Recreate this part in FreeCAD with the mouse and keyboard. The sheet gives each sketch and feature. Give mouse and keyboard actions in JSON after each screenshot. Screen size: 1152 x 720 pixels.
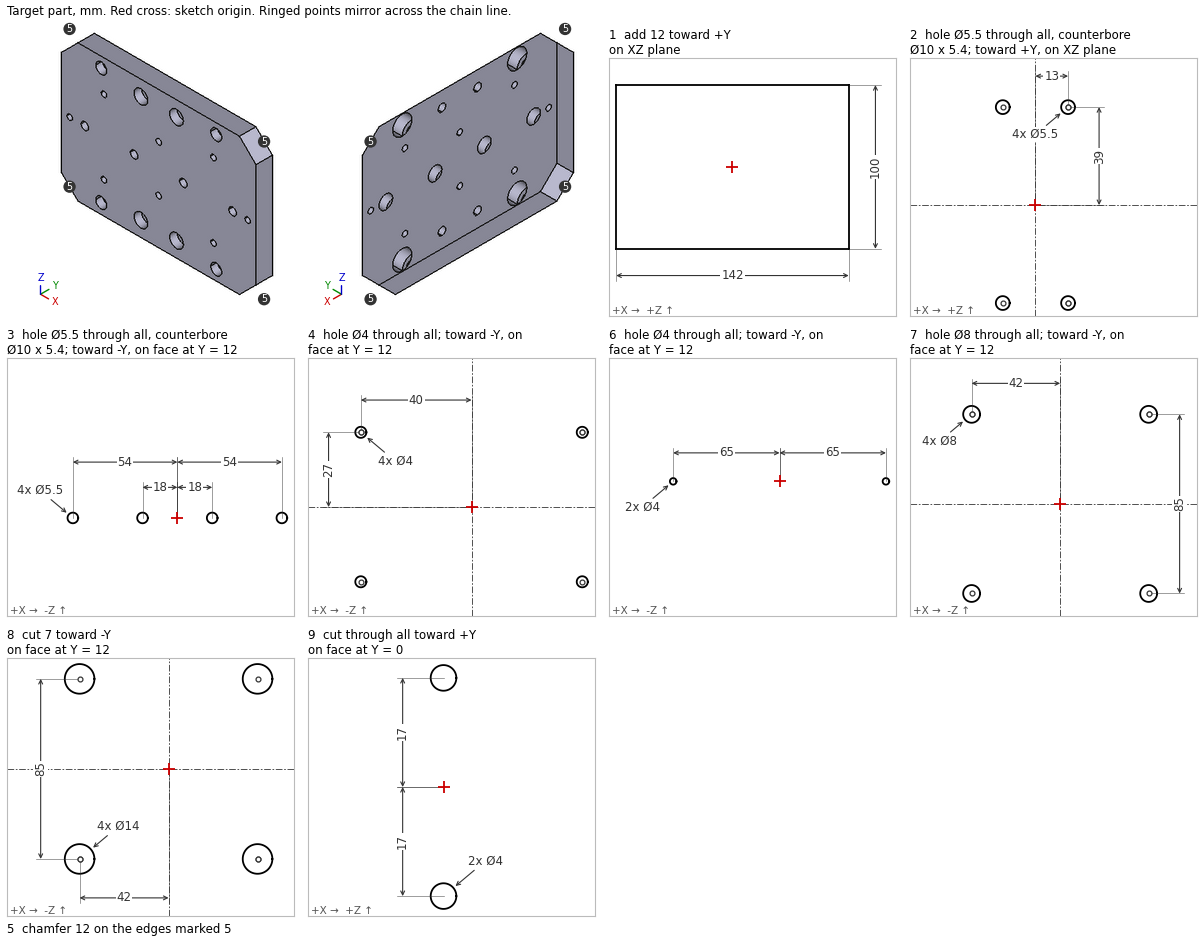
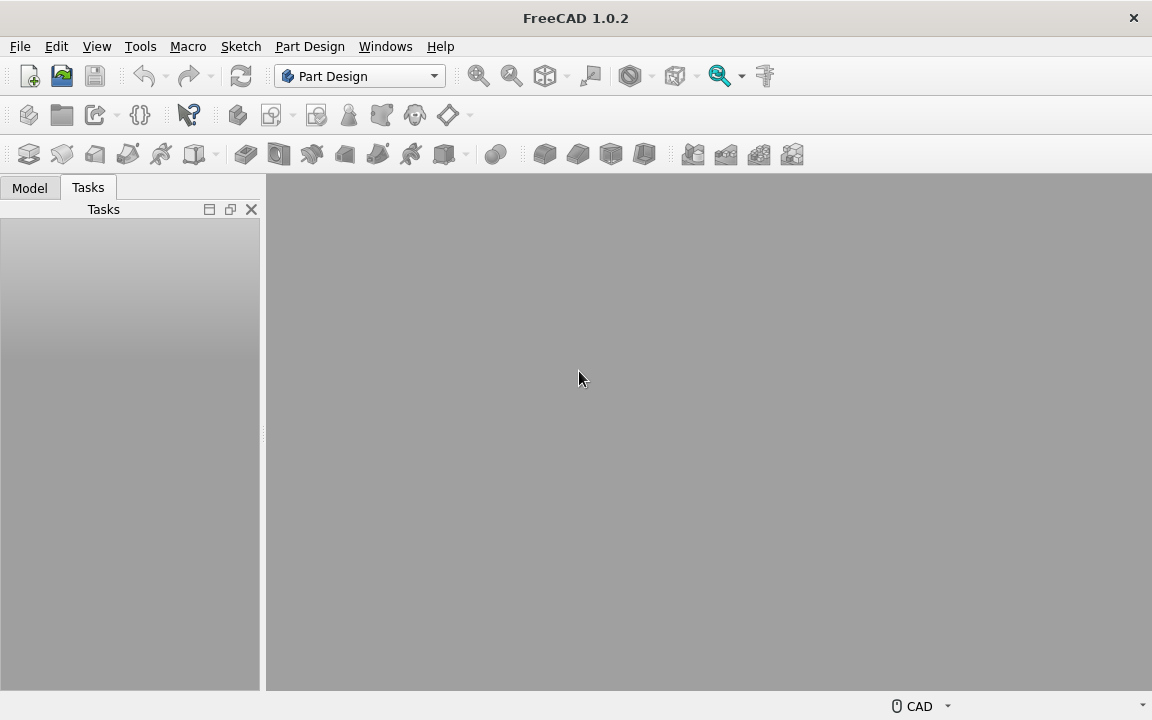
{"action": "left_click", "coordinate": [29, 76]}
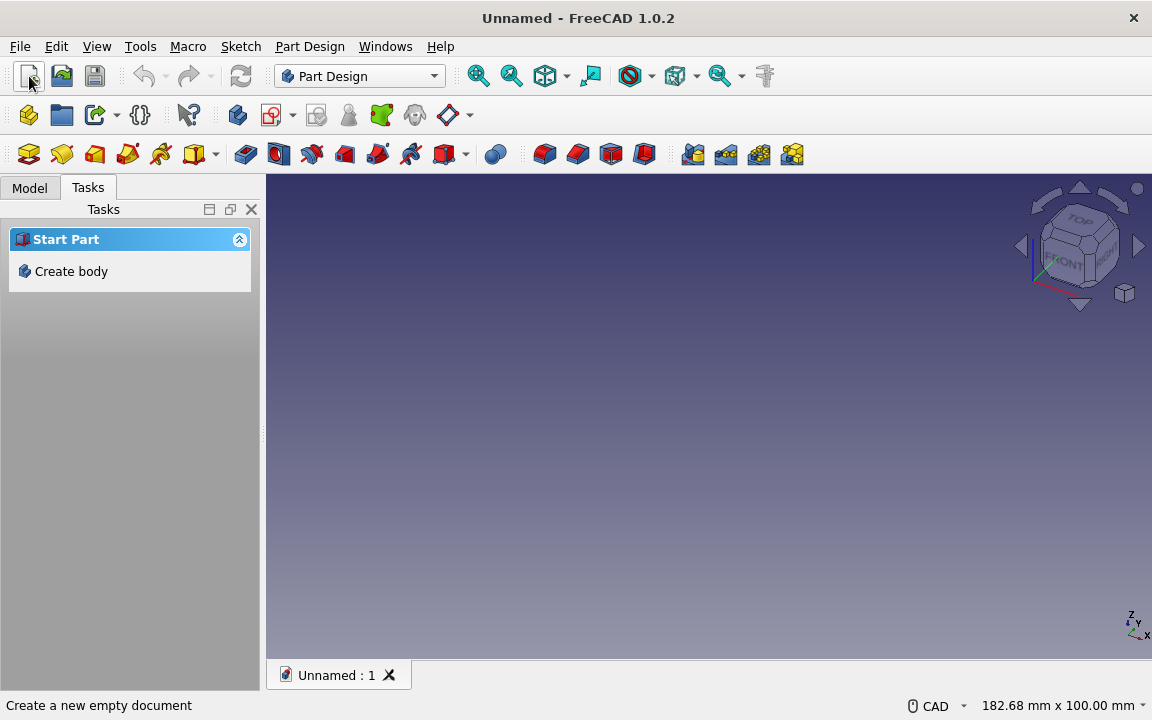
{"action": "left_click", "coordinate": [270, 116]}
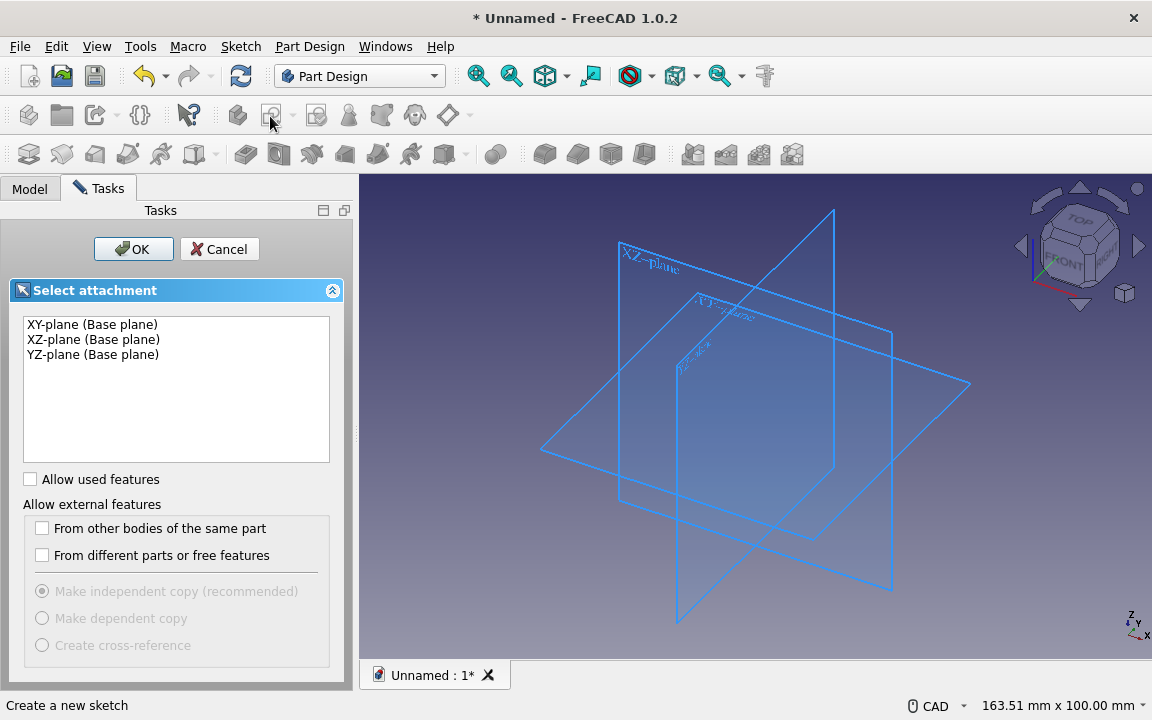
{"action": "left_click", "coordinate": [84, 340]}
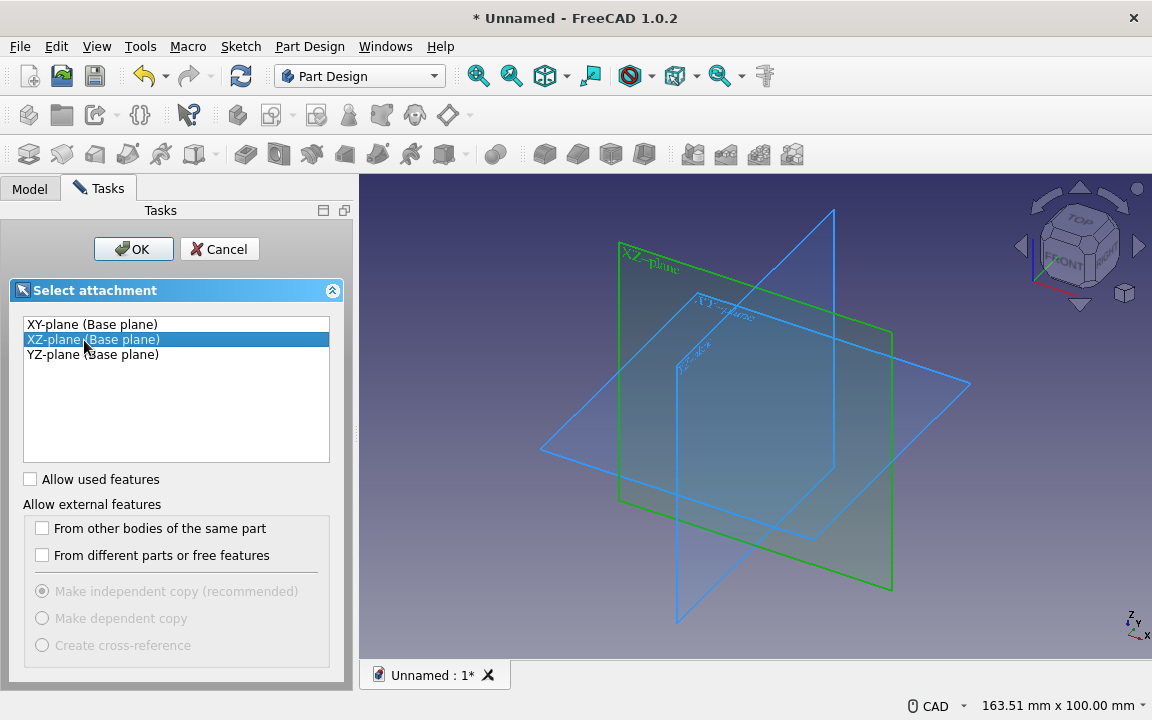
{"action": "left_click", "coordinate": [134, 249]}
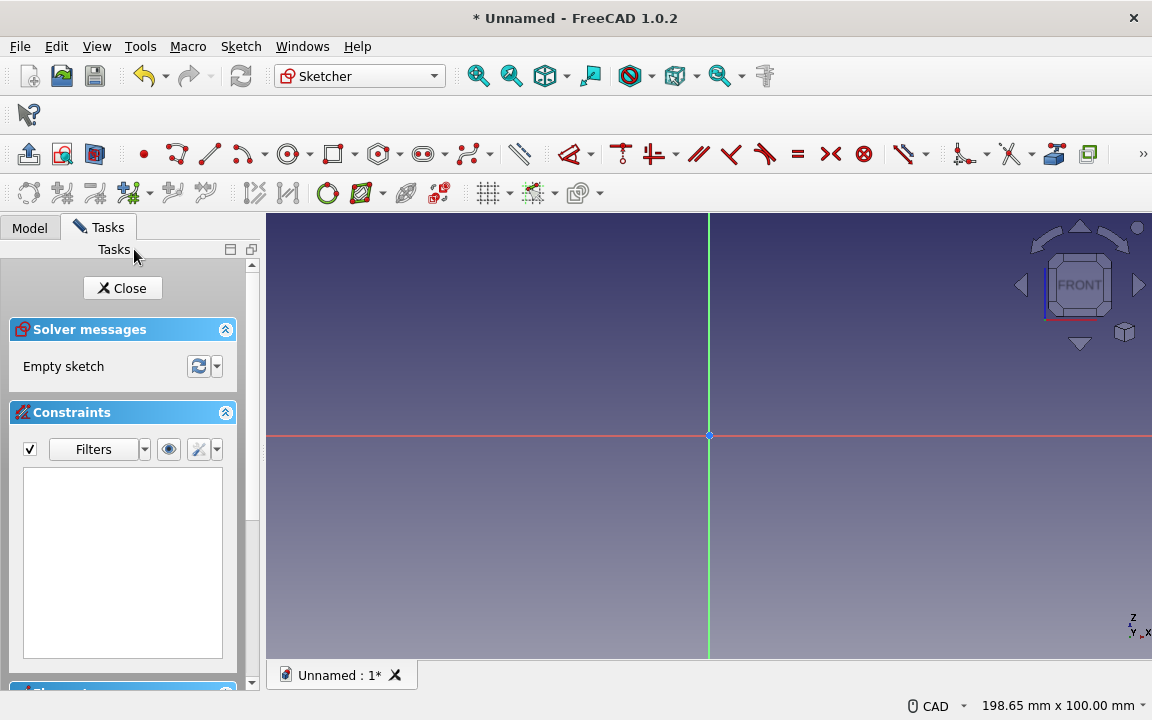
{"action": "scroll", "coordinate": [501, 436], "scroll_direction": "down", "scroll_amount": 2}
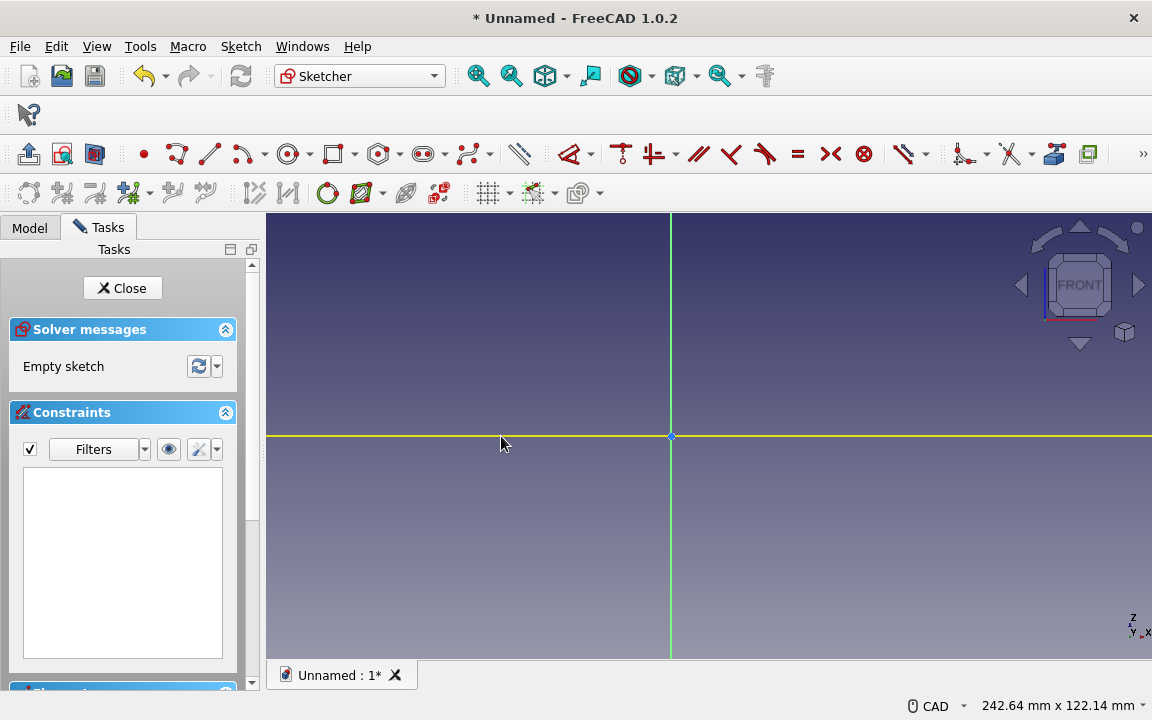
{"action": "left_click", "coordinate": [354, 154]}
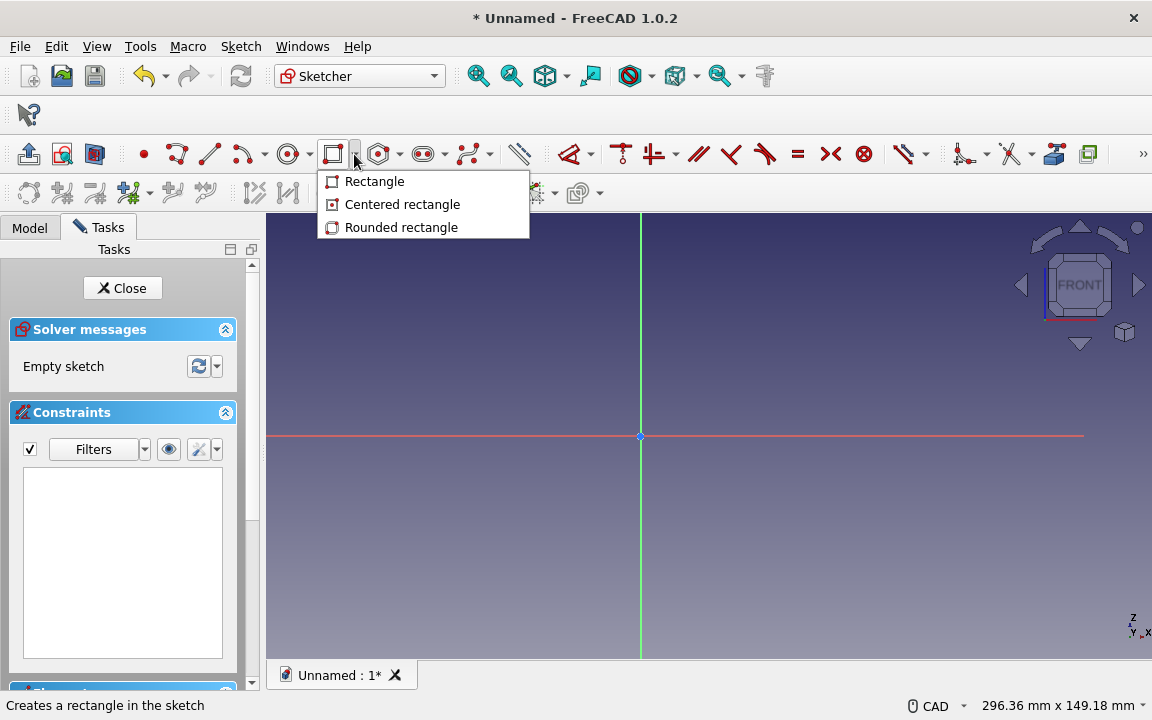
{"action": "left_click", "coordinate": [424, 204]}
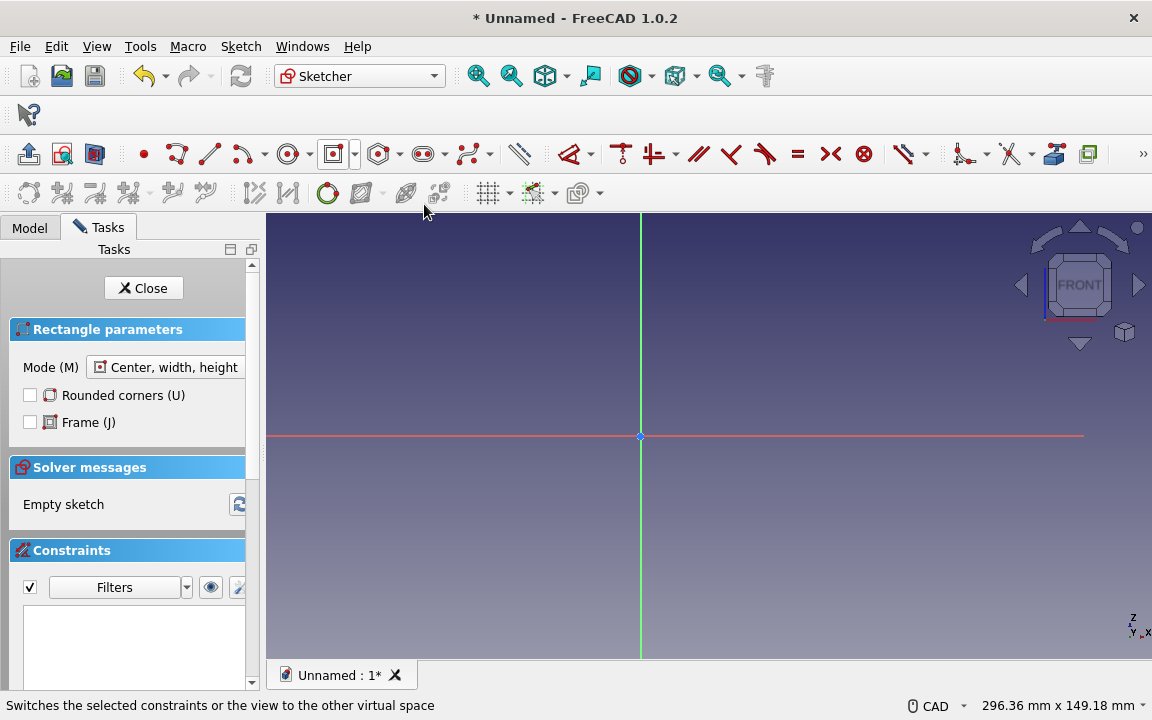
{"action": "left_click", "coordinate": [641, 436]}
{"action": "left_click", "coordinate": [853, 287]}
{"action": "key", "text": "Escape"}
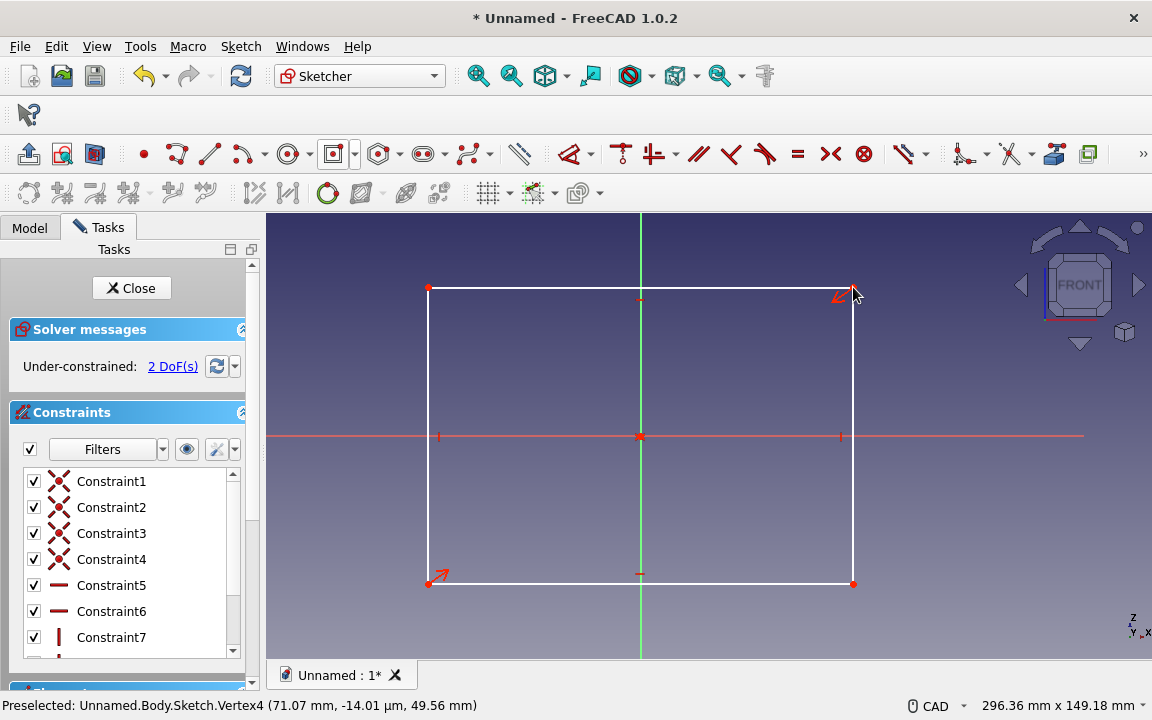
{"action": "left_click", "coordinate": [568, 154]}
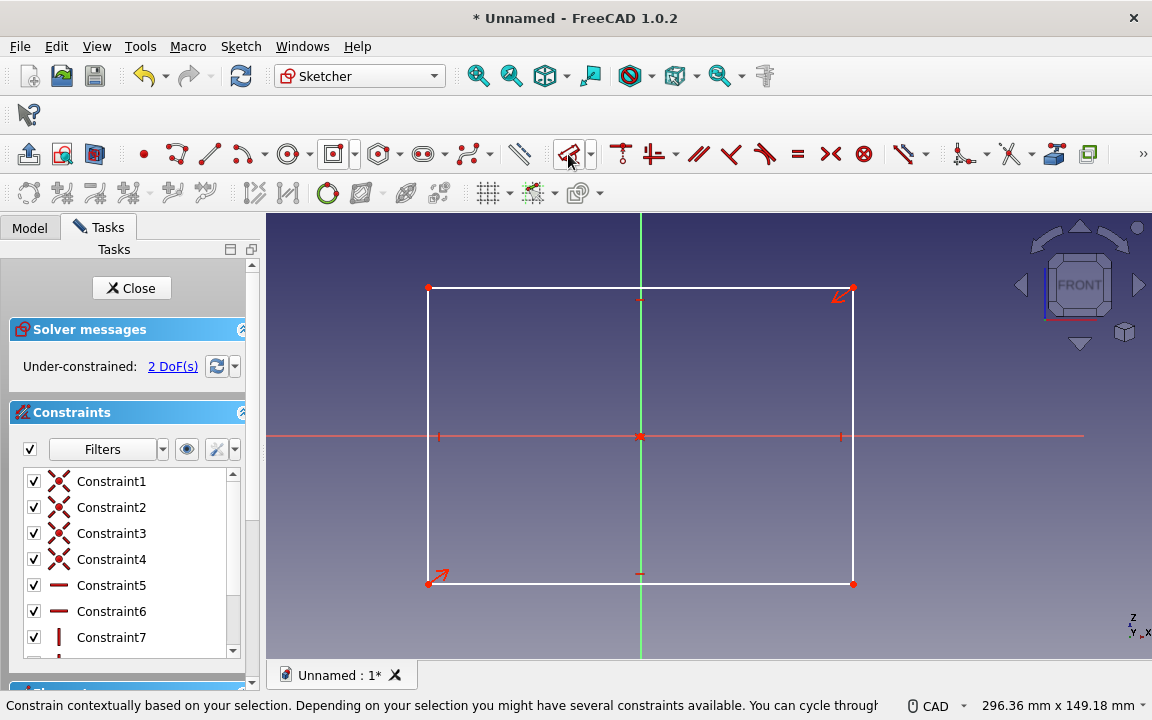
{"action": "left_click", "coordinate": [556, 584]}
{"action": "left_click", "coordinate": [543, 618]}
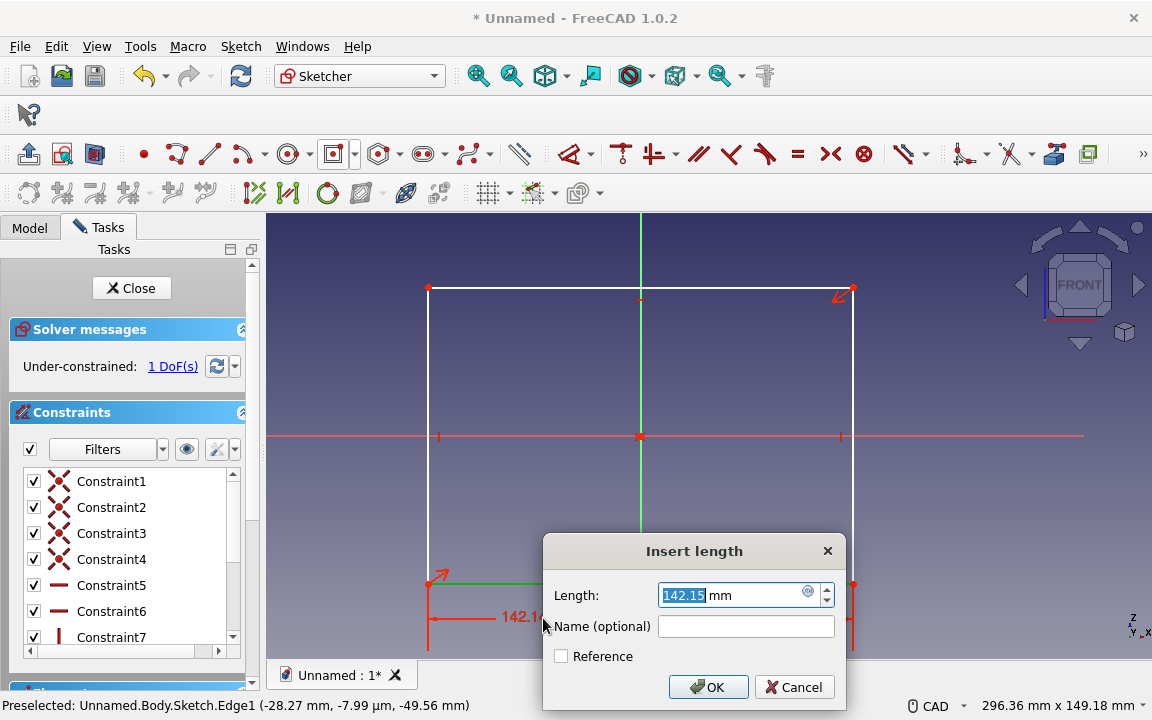
{"action": "type", "text": "142"}
{"action": "key", "text": "Return"}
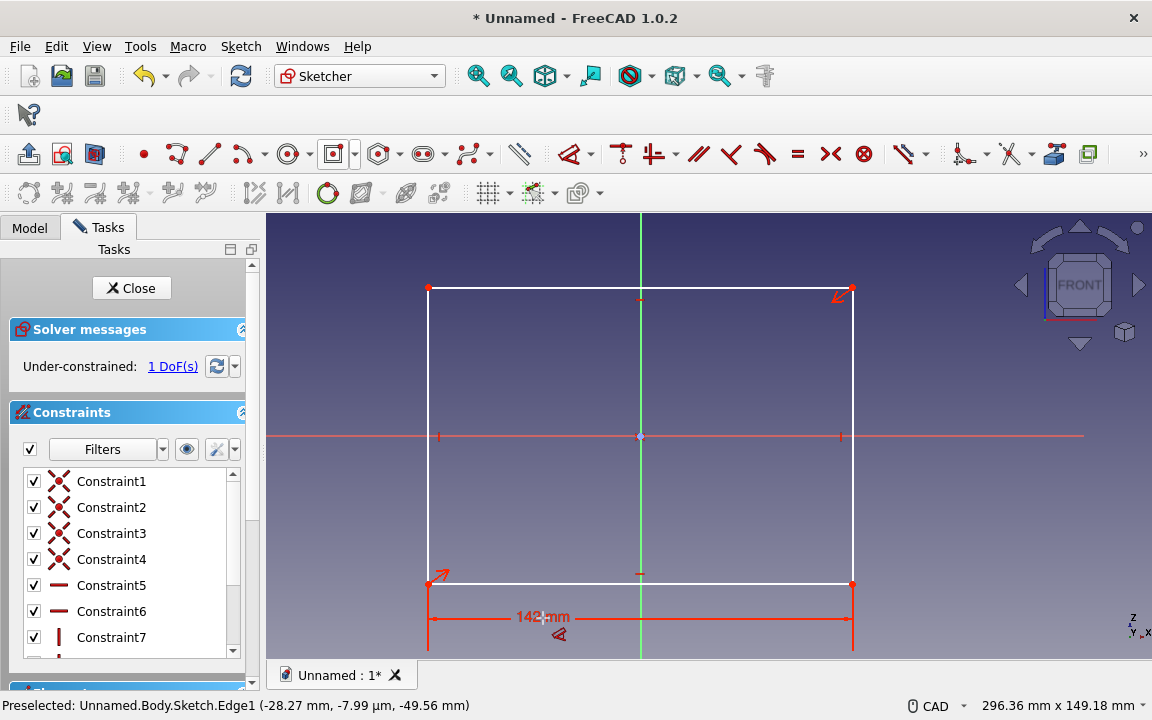
{"action": "left_click", "coordinate": [853, 495]}
{"action": "left_click", "coordinate": [887, 368]}